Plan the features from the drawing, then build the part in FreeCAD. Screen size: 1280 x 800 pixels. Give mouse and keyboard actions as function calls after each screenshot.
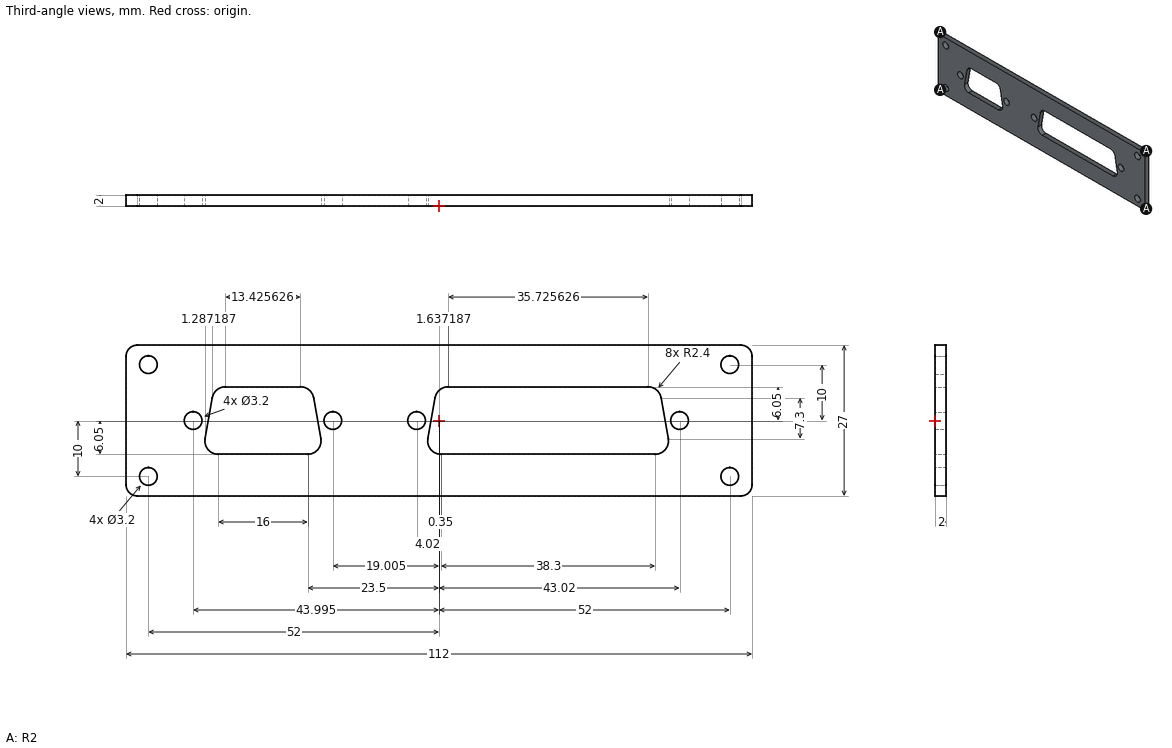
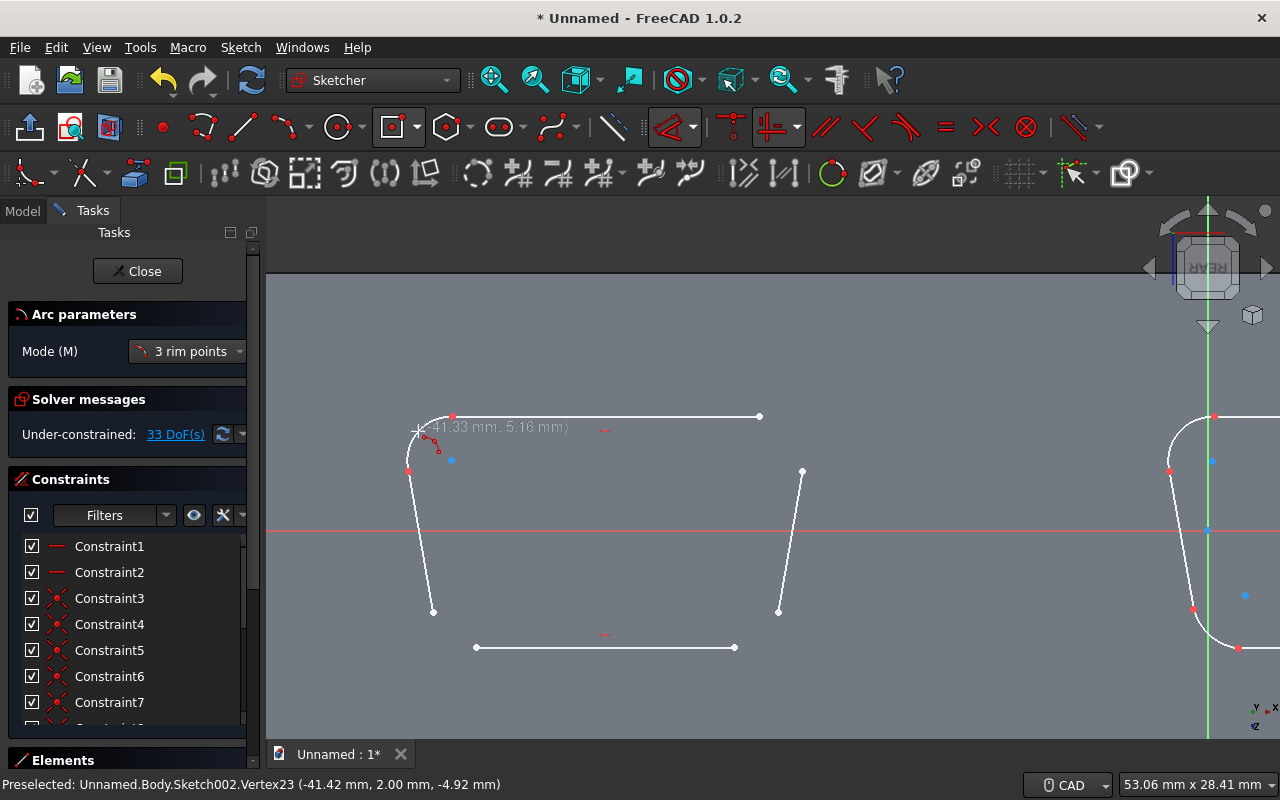
click(433, 612)
click(477, 648)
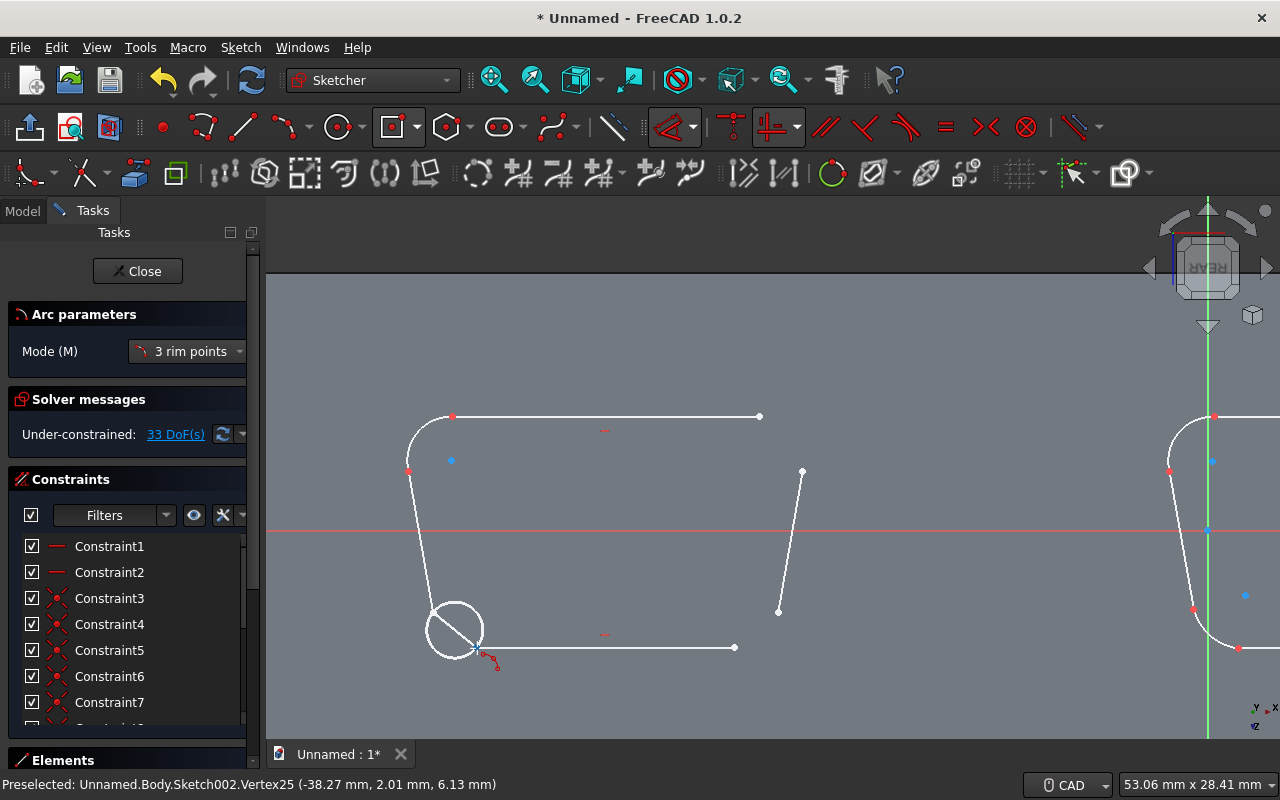
scroll(448, 636, up, 2)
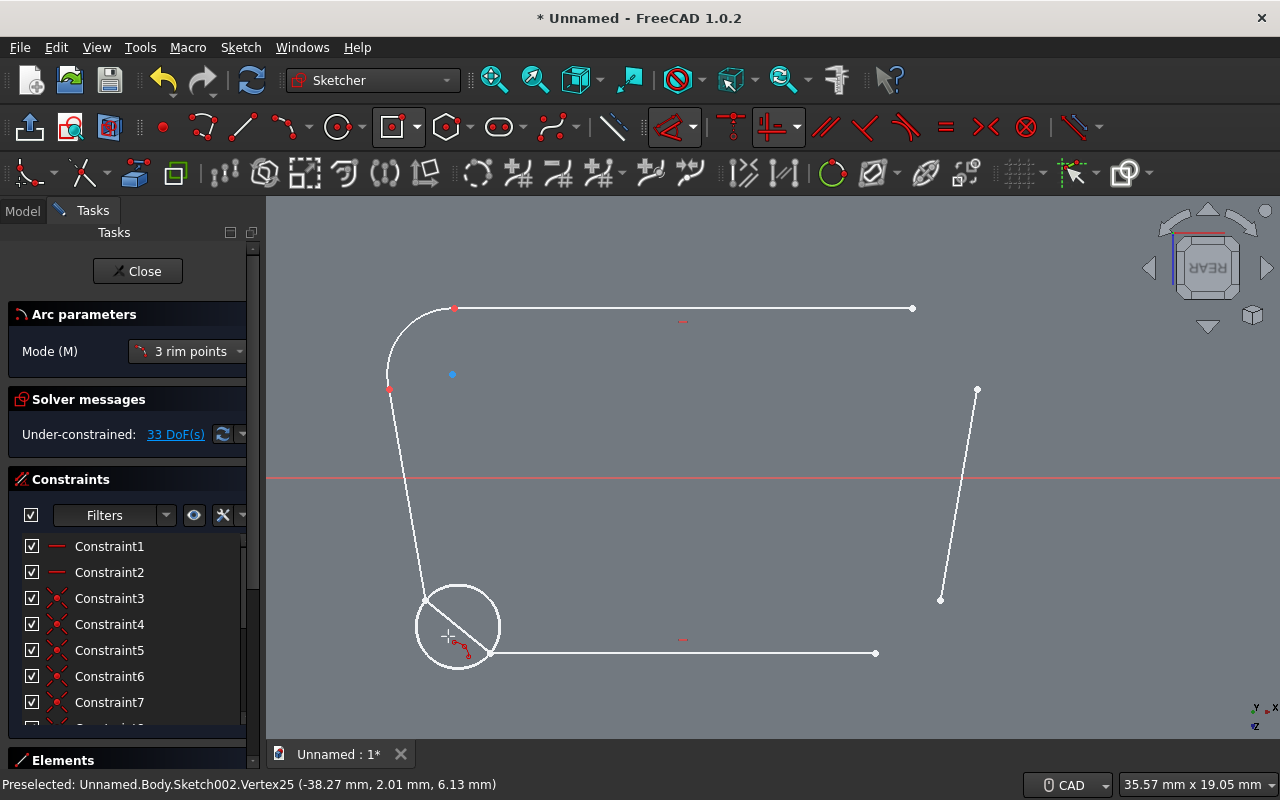
click(448, 635)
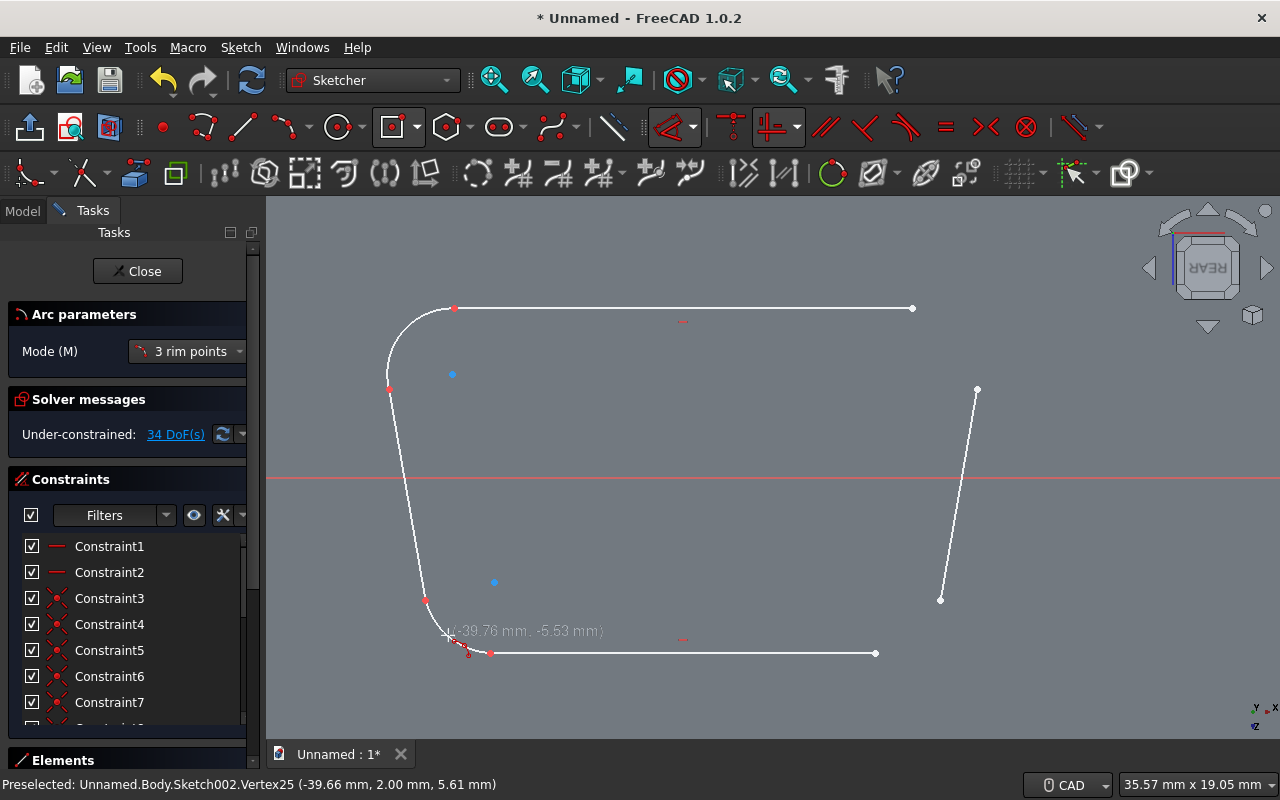
scroll(422, 464, down, 7)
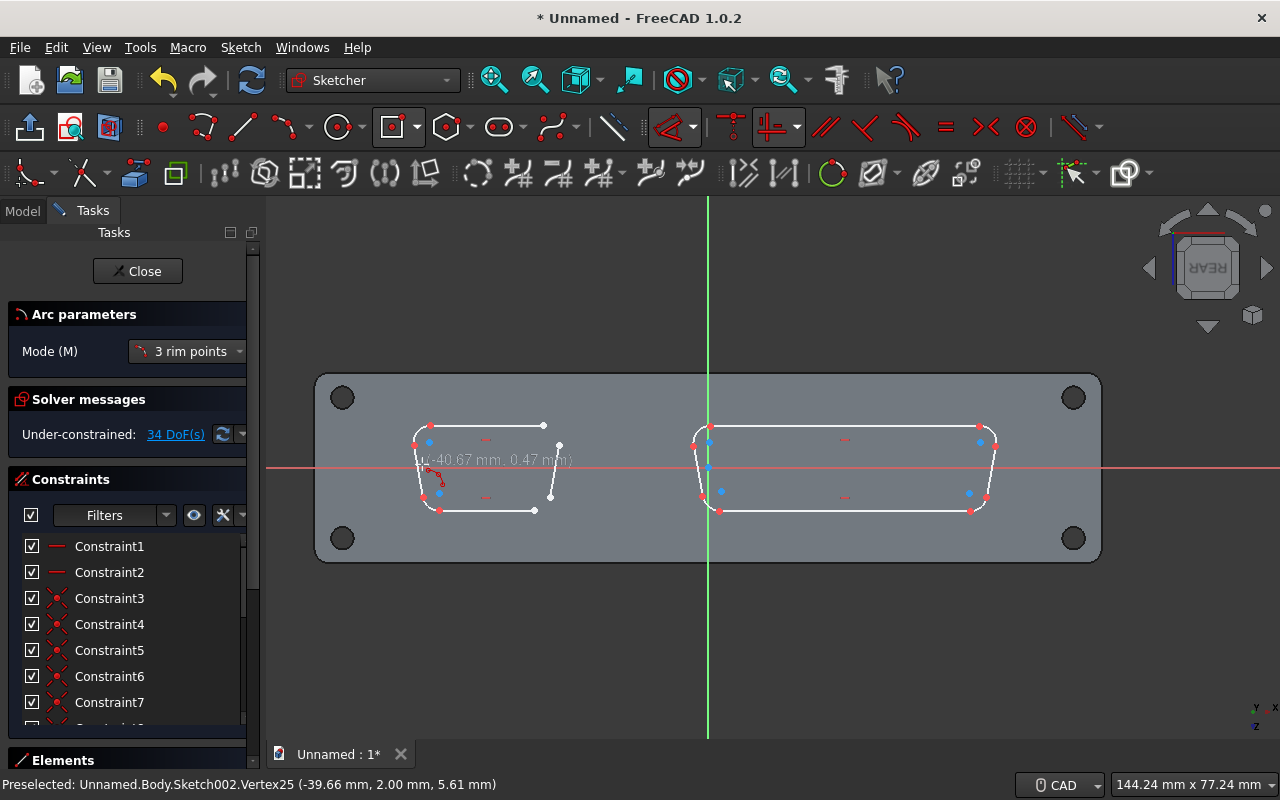
click(534, 511)
click(550, 498)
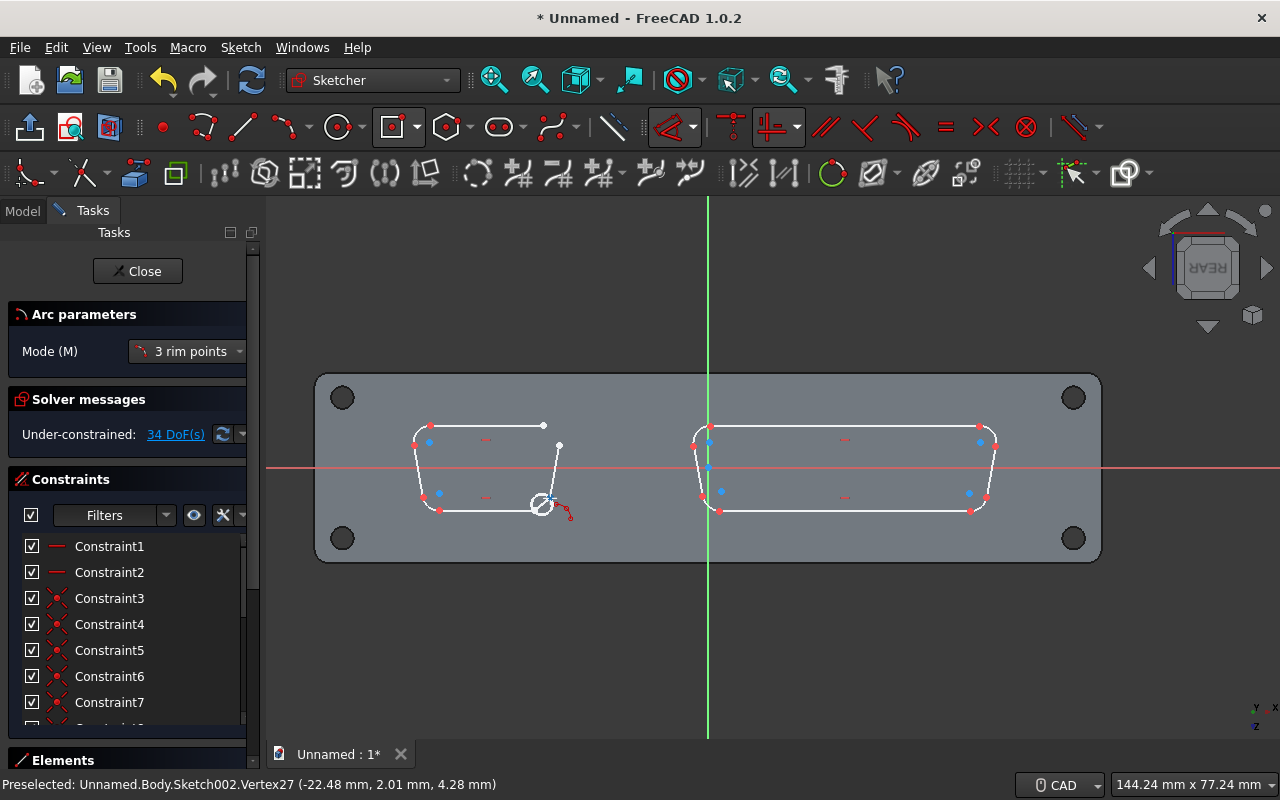
scroll(545, 507, up, 7)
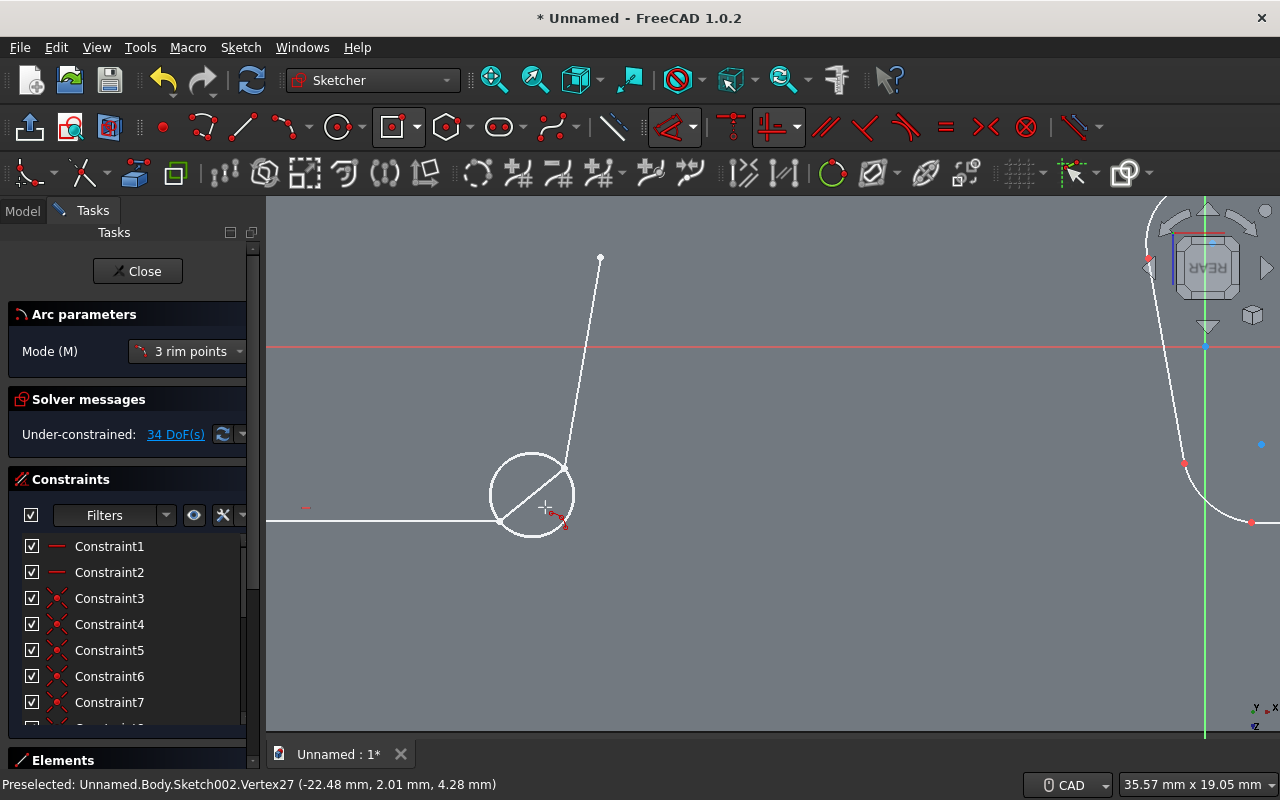
click(543, 503)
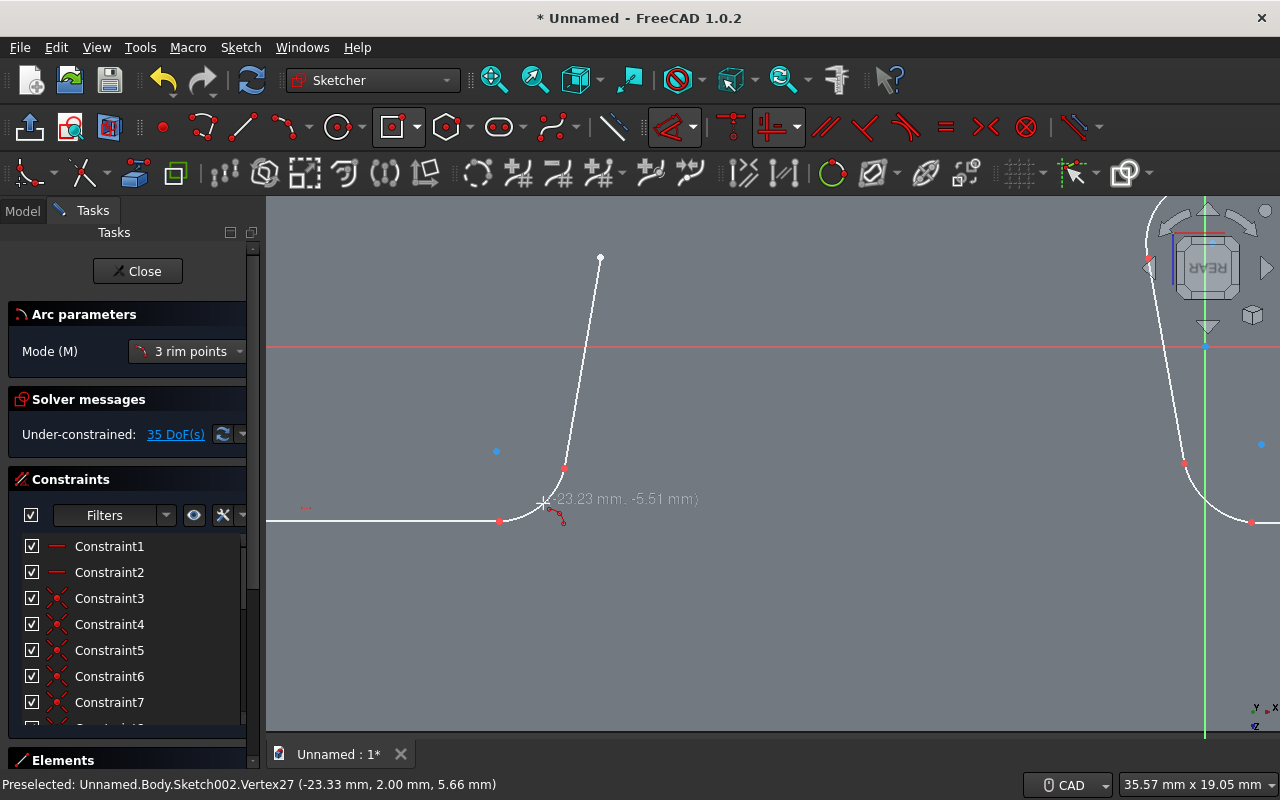
scroll(545, 507, down, 7)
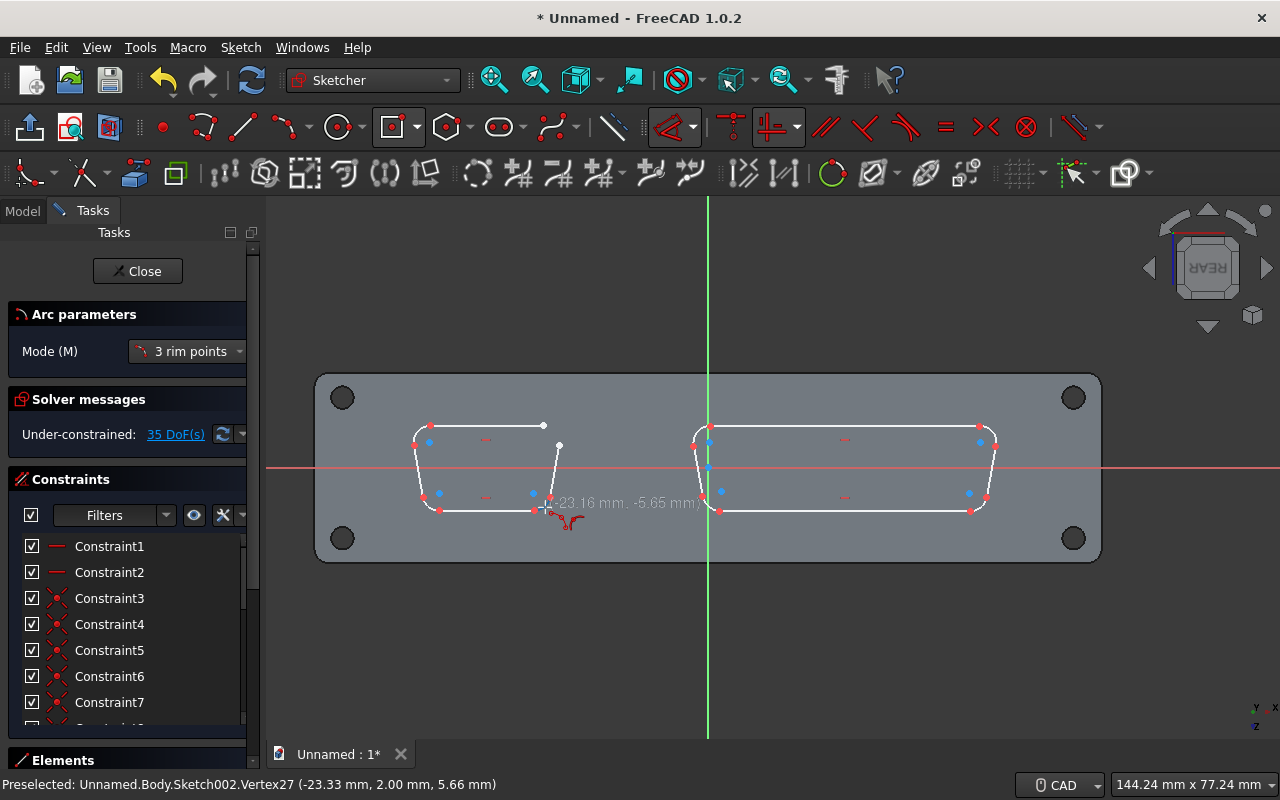
click(559, 446)
click(543, 426)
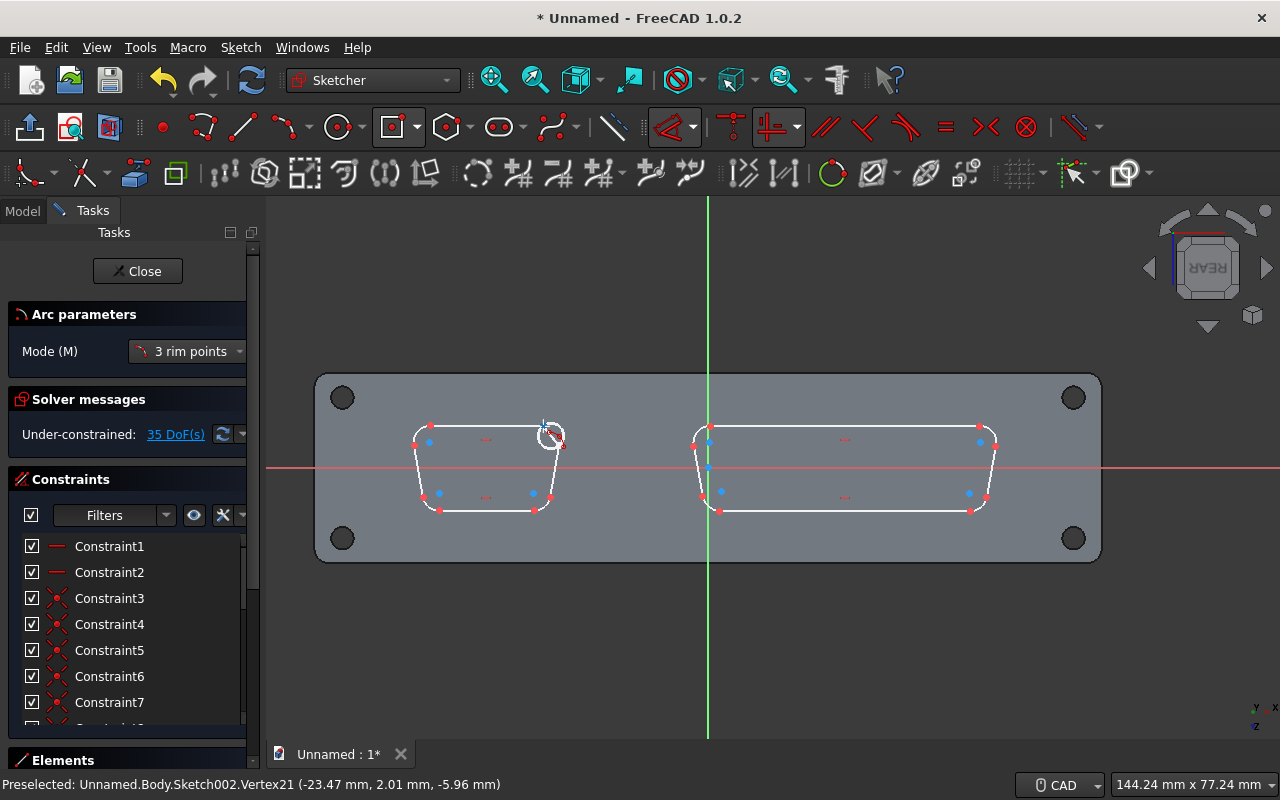
scroll(556, 431, up, 5)